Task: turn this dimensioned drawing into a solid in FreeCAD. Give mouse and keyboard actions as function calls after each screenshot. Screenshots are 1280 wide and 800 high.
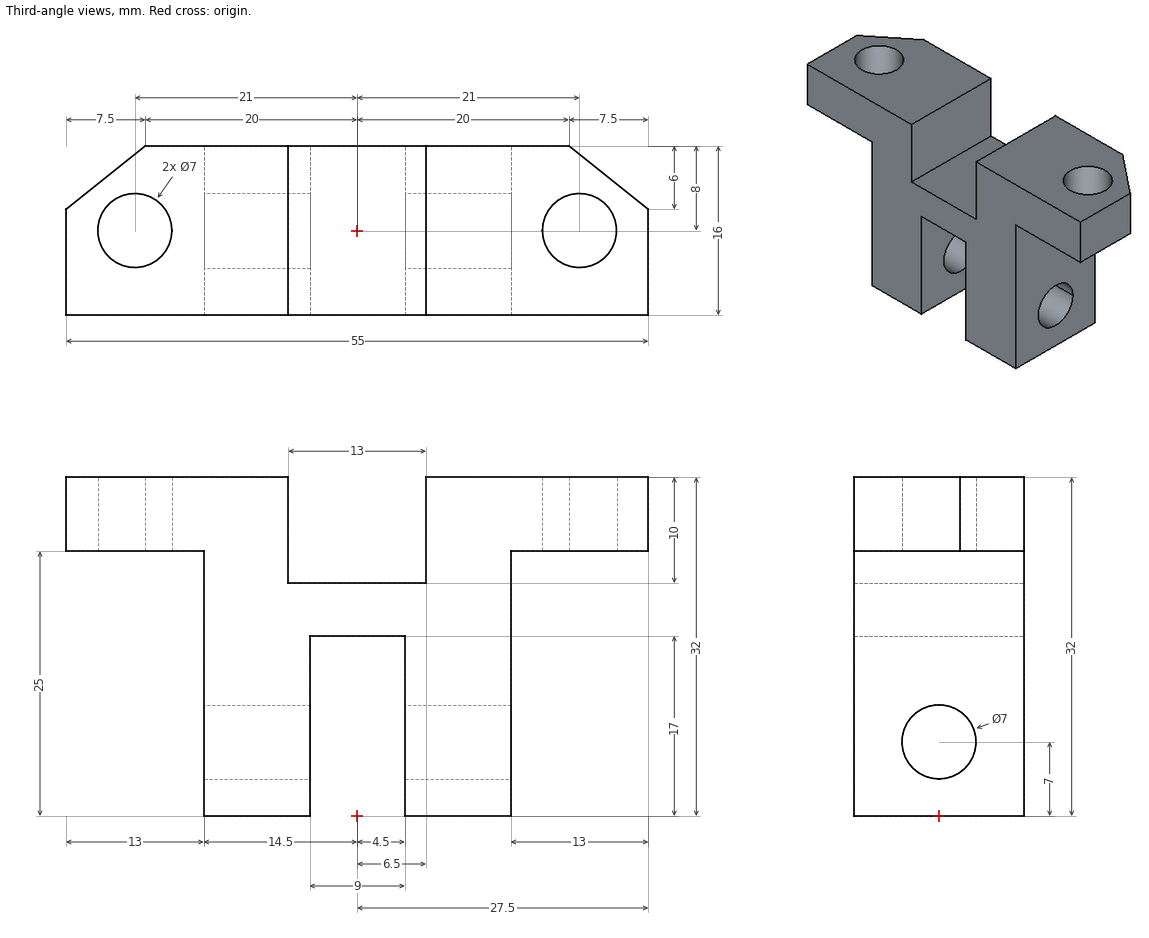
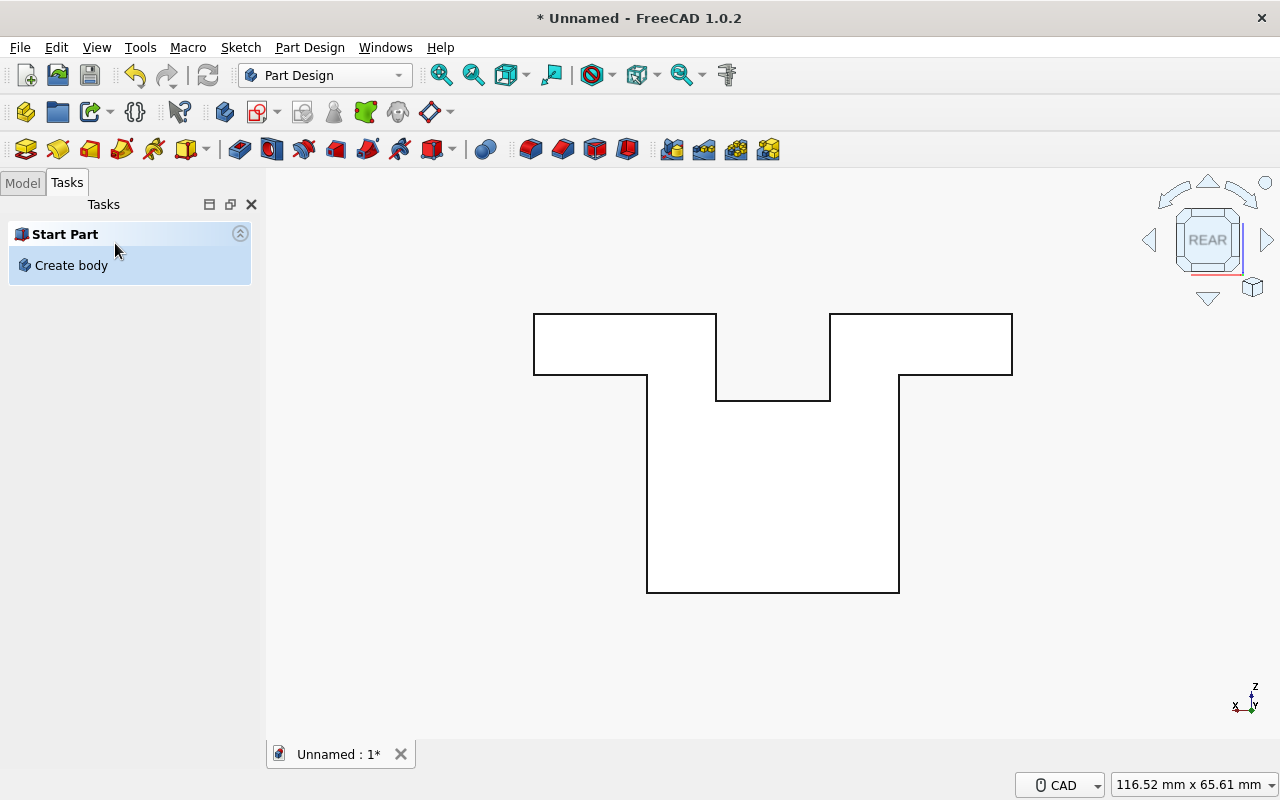
click(773, 492)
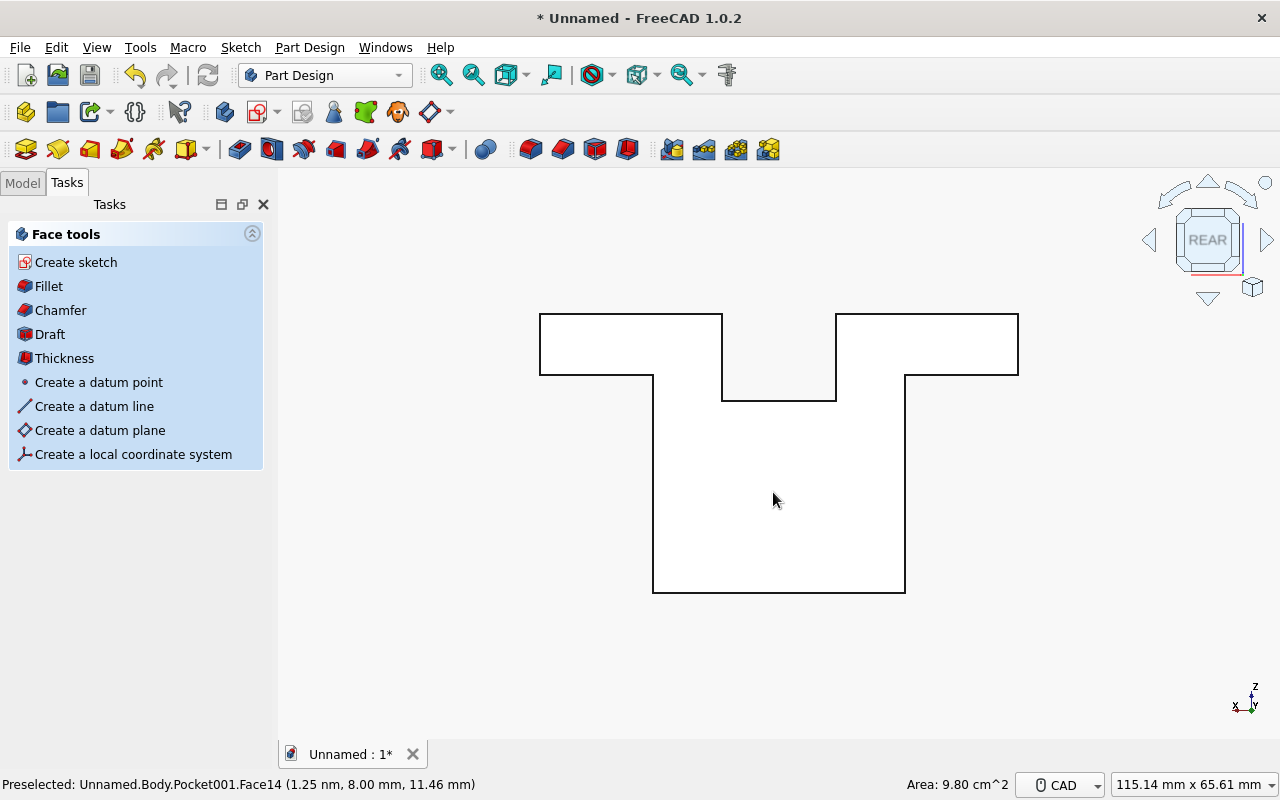
click(258, 112)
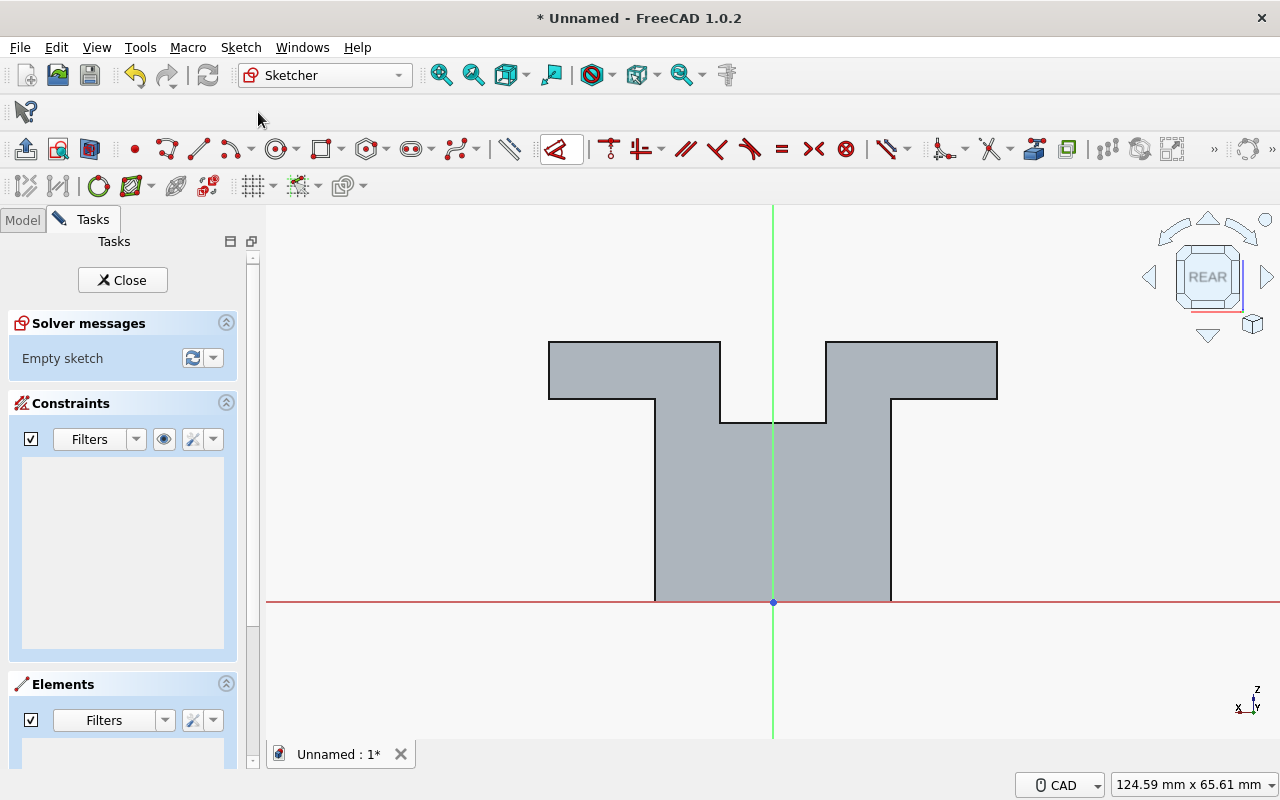
scroll(829, 583, up, 4)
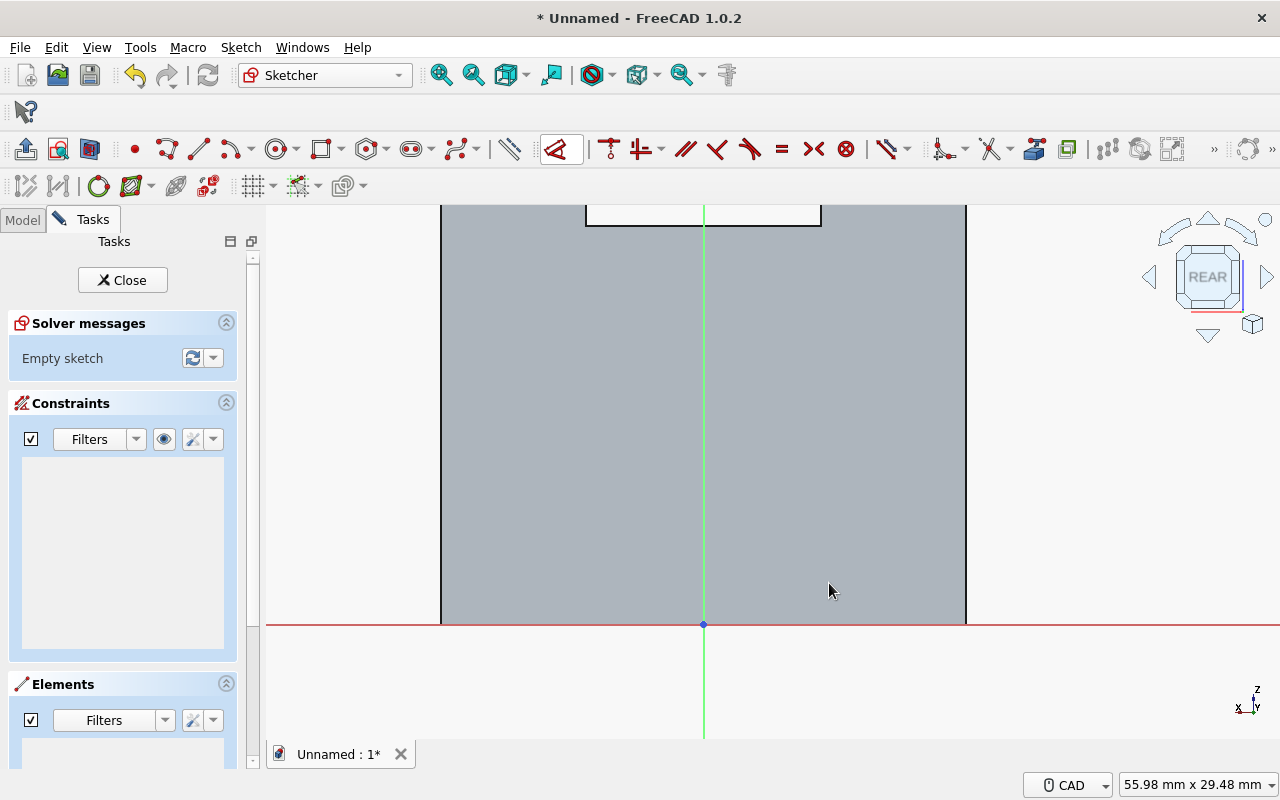
click(322, 150)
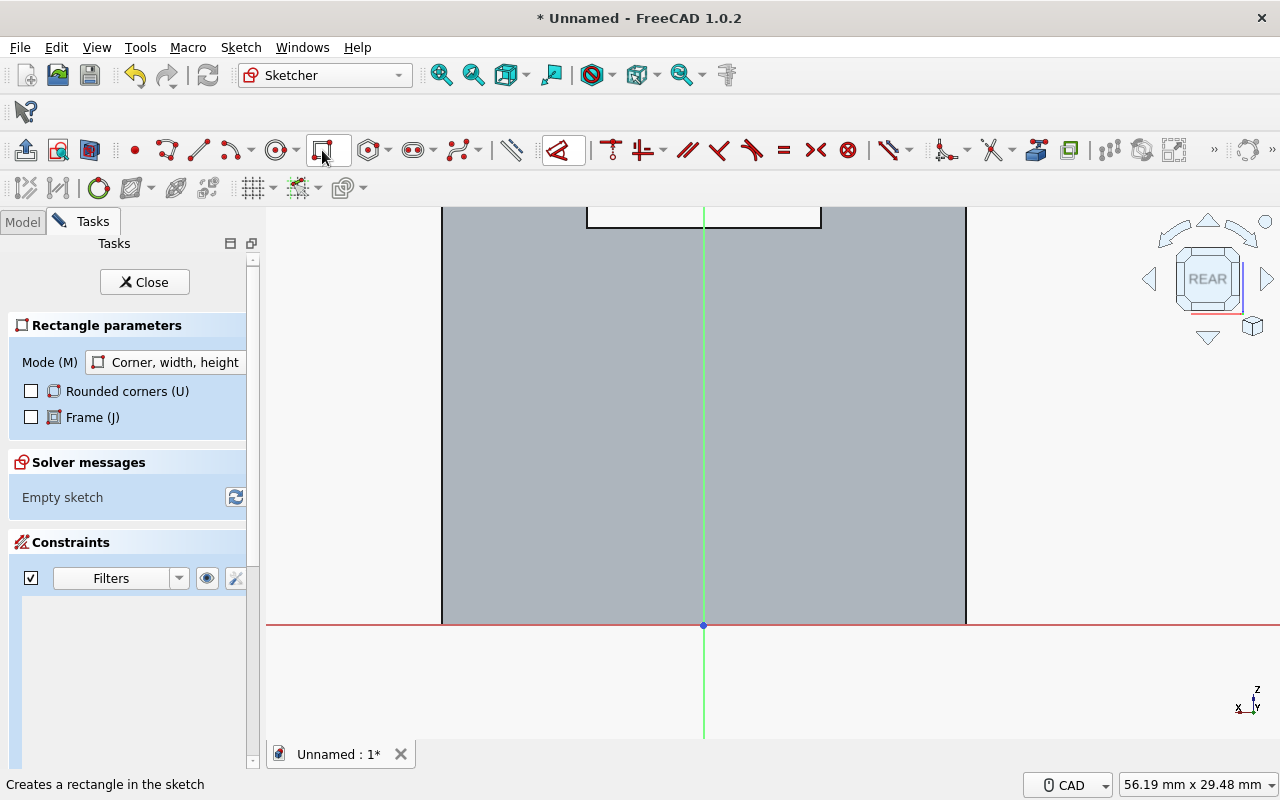
click(623, 319)
click(785, 625)
key(Escape)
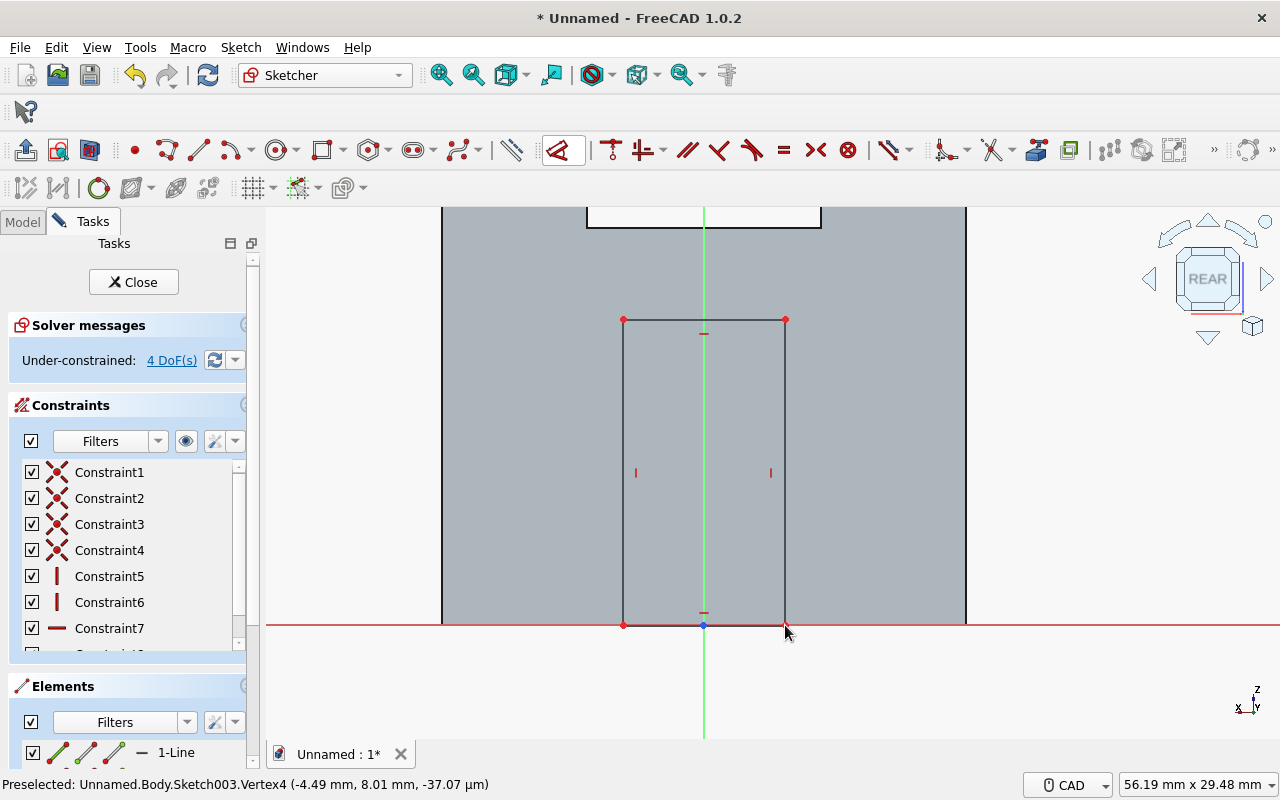
click(623, 626)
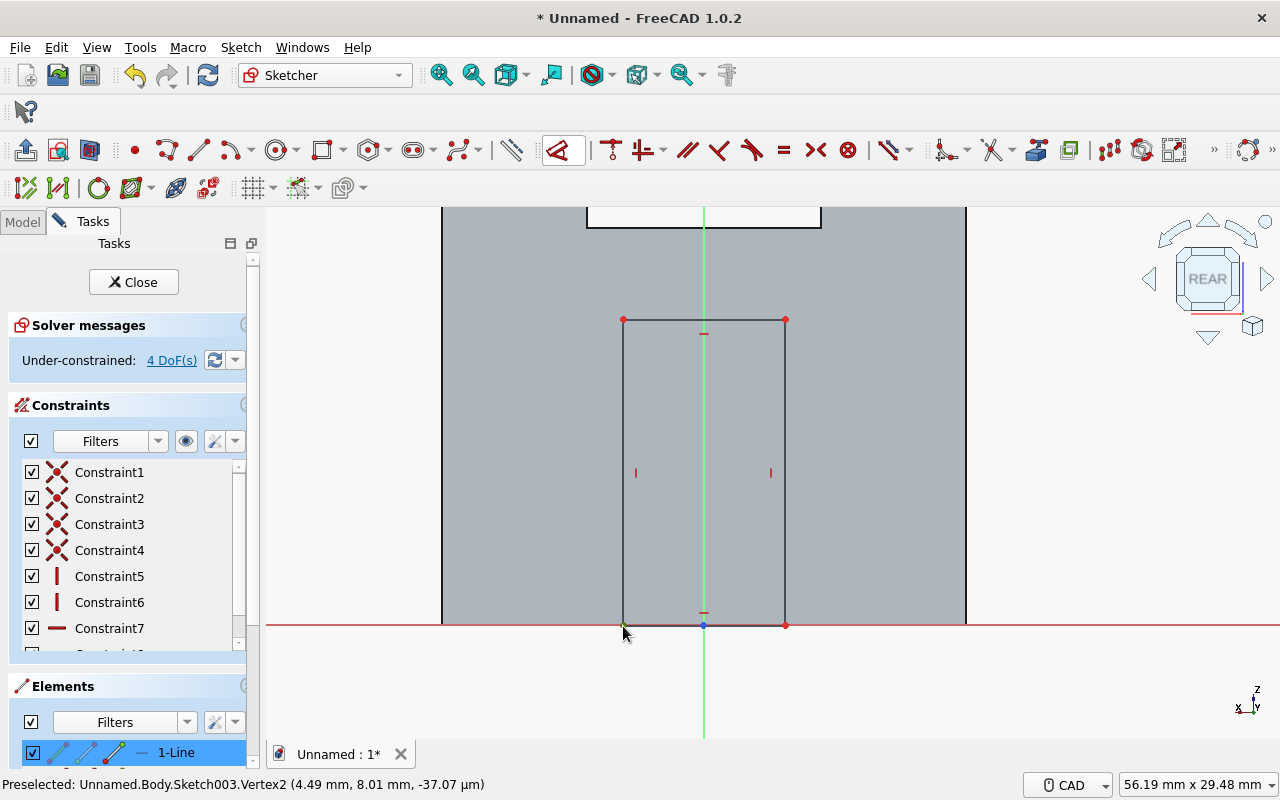
click(353, 625)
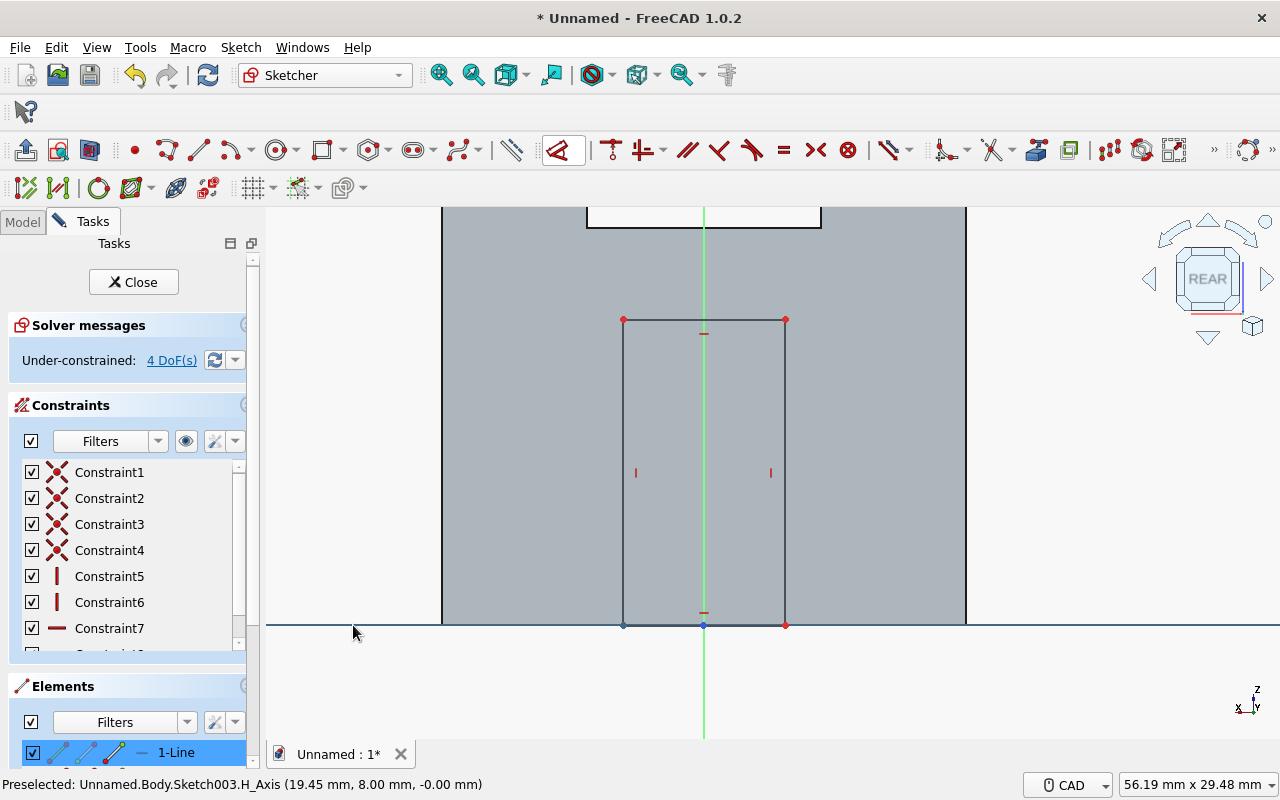
key(c)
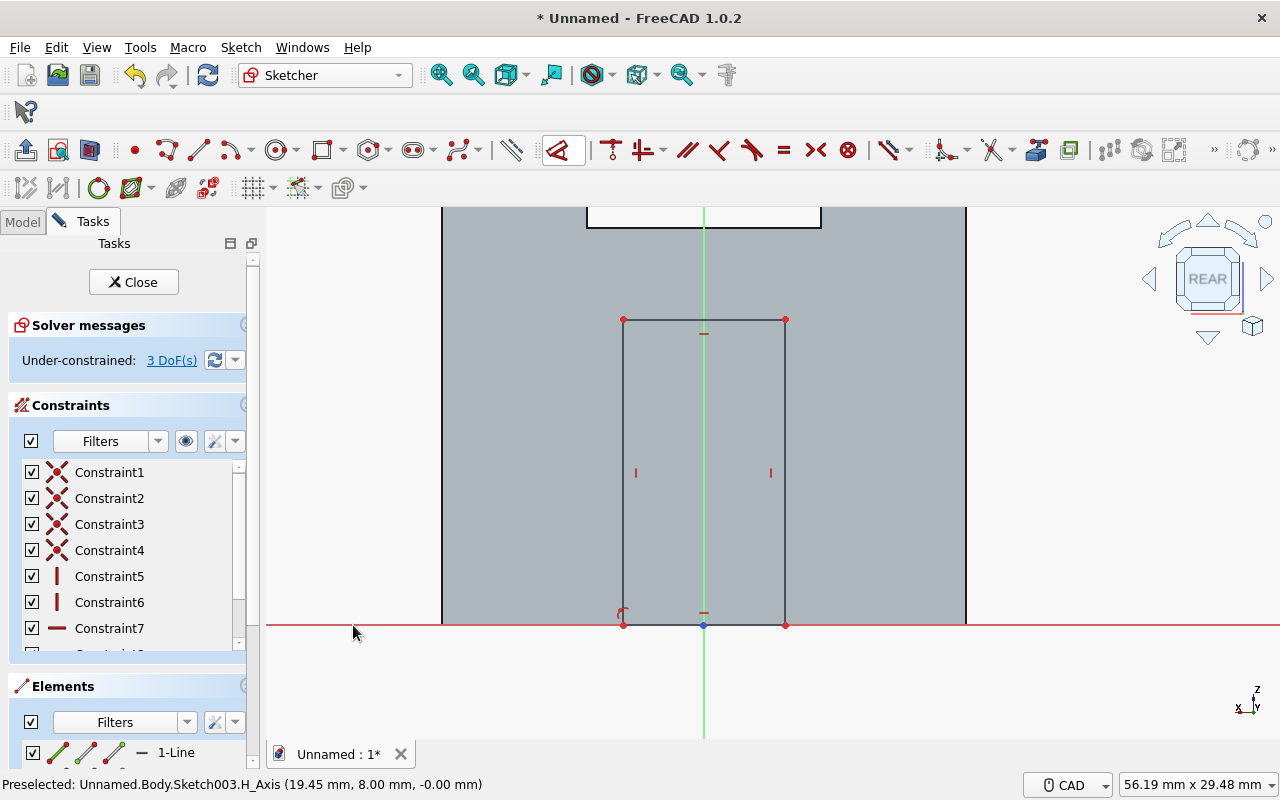
click(672, 625)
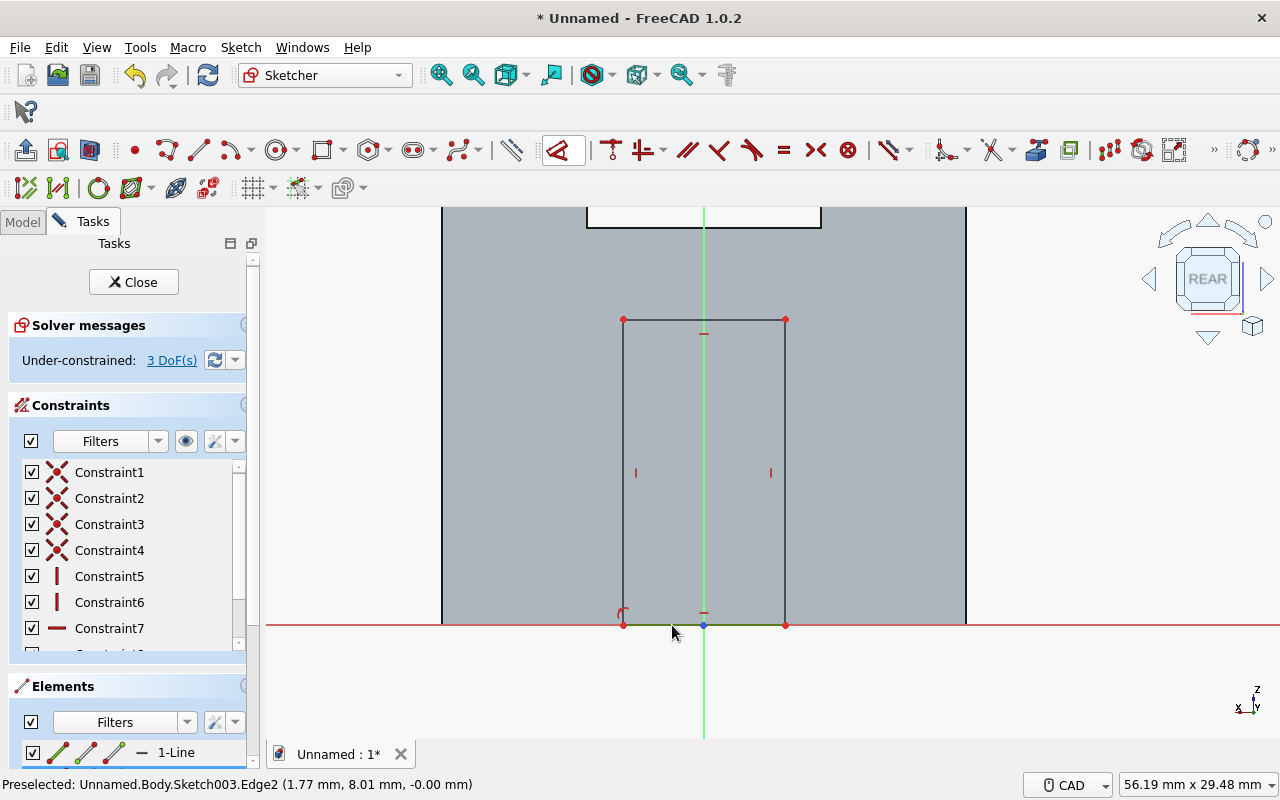
click(580, 150)